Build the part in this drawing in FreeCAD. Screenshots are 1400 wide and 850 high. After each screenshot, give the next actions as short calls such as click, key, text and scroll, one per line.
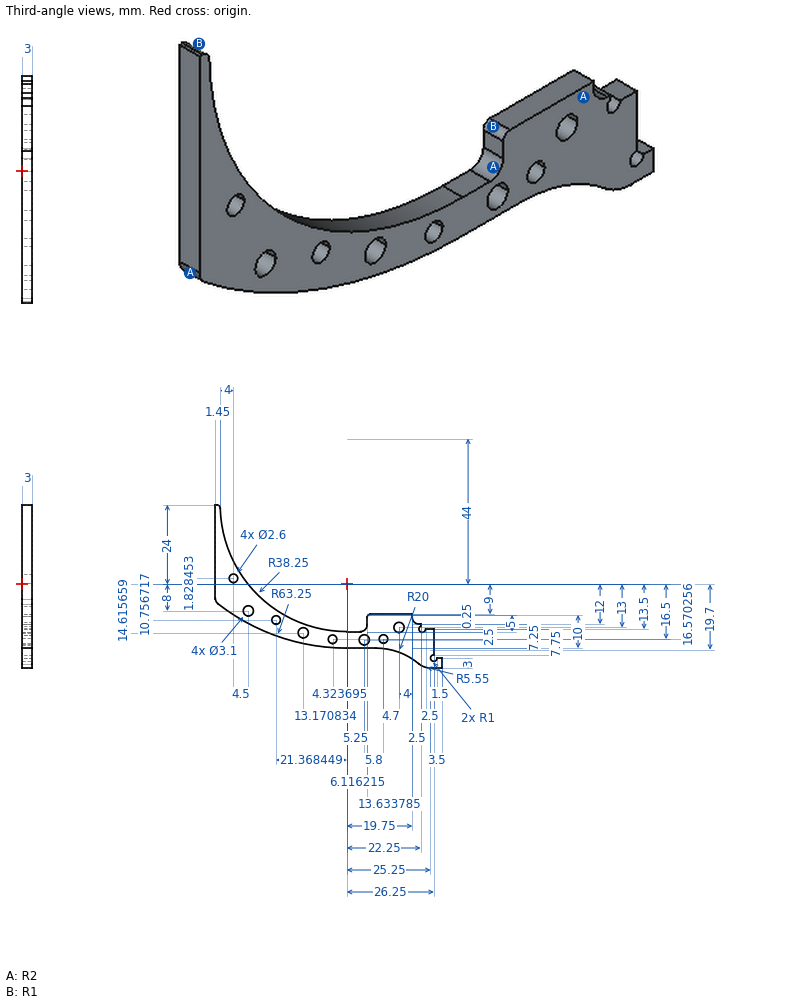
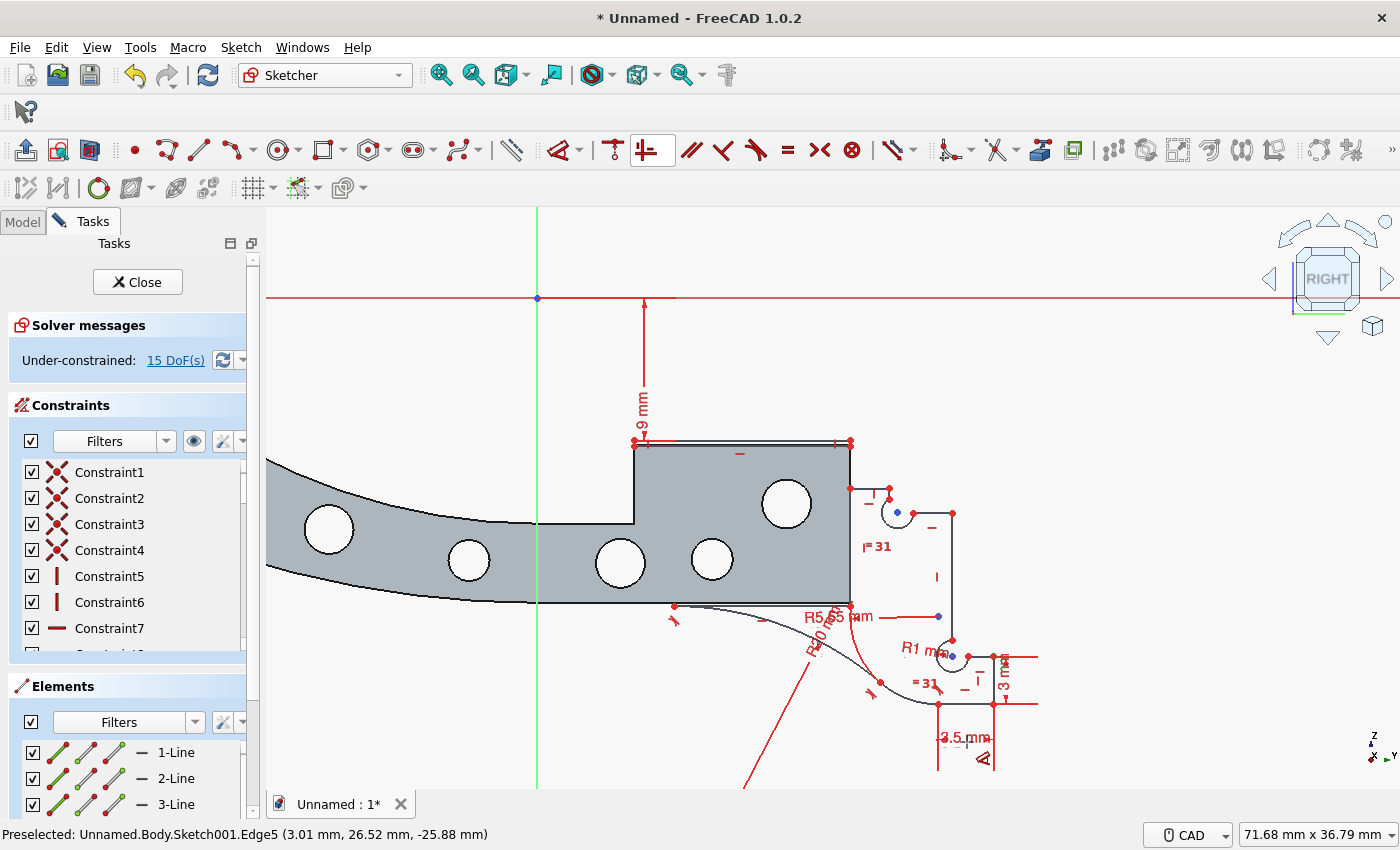
scroll(983, 657, up, 3)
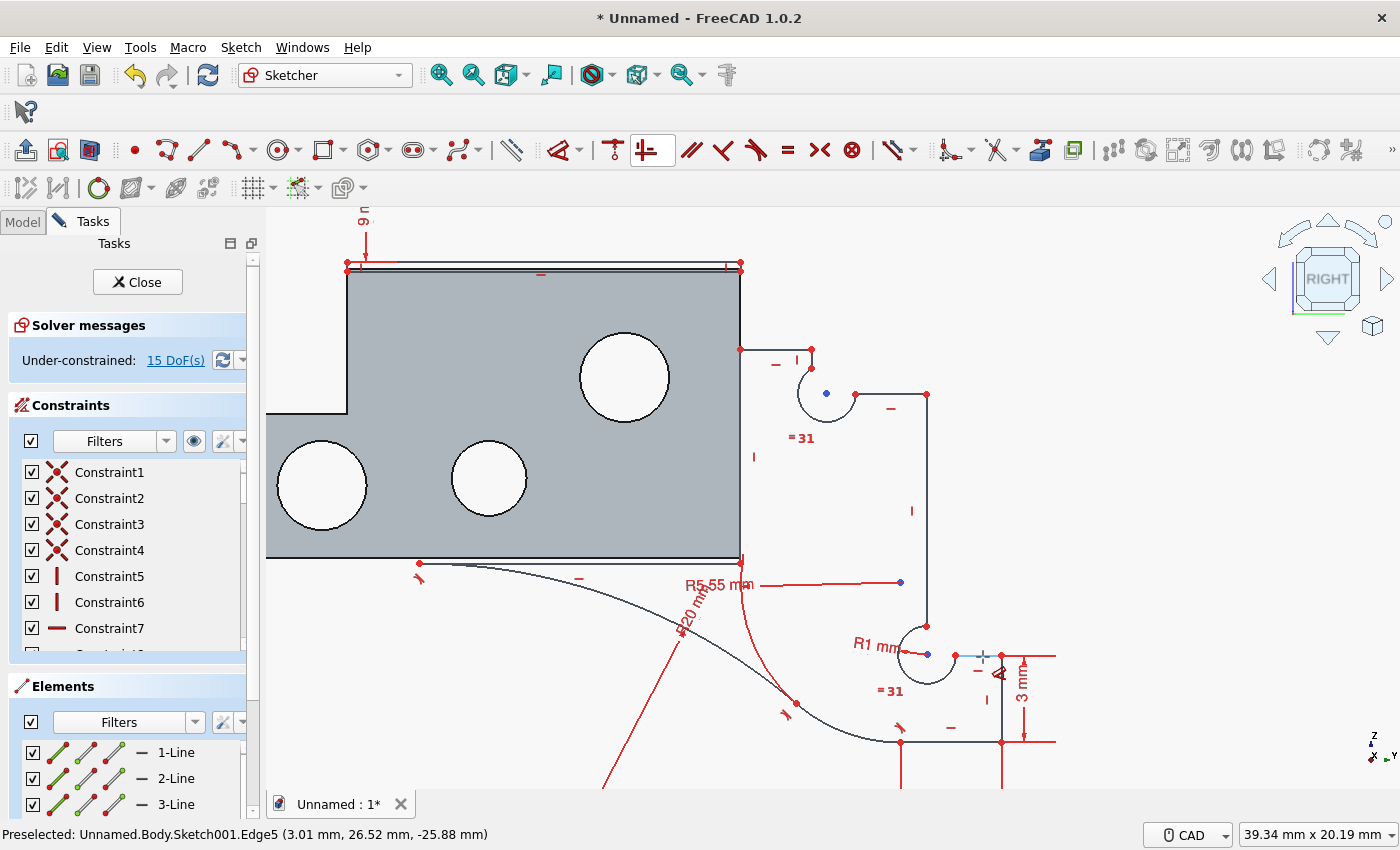
click(983, 656)
click(979, 622)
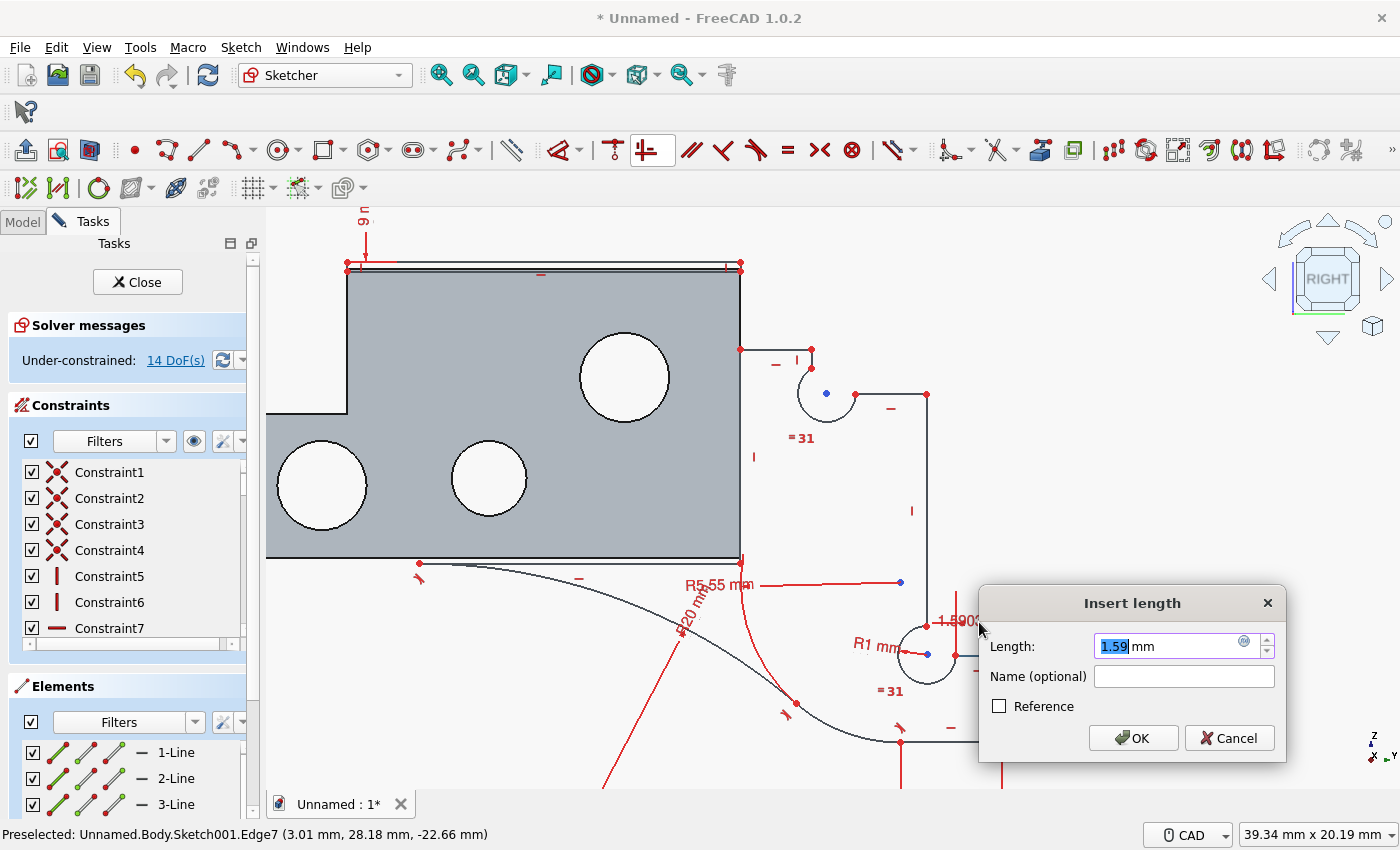
text(1.5)
key(Return)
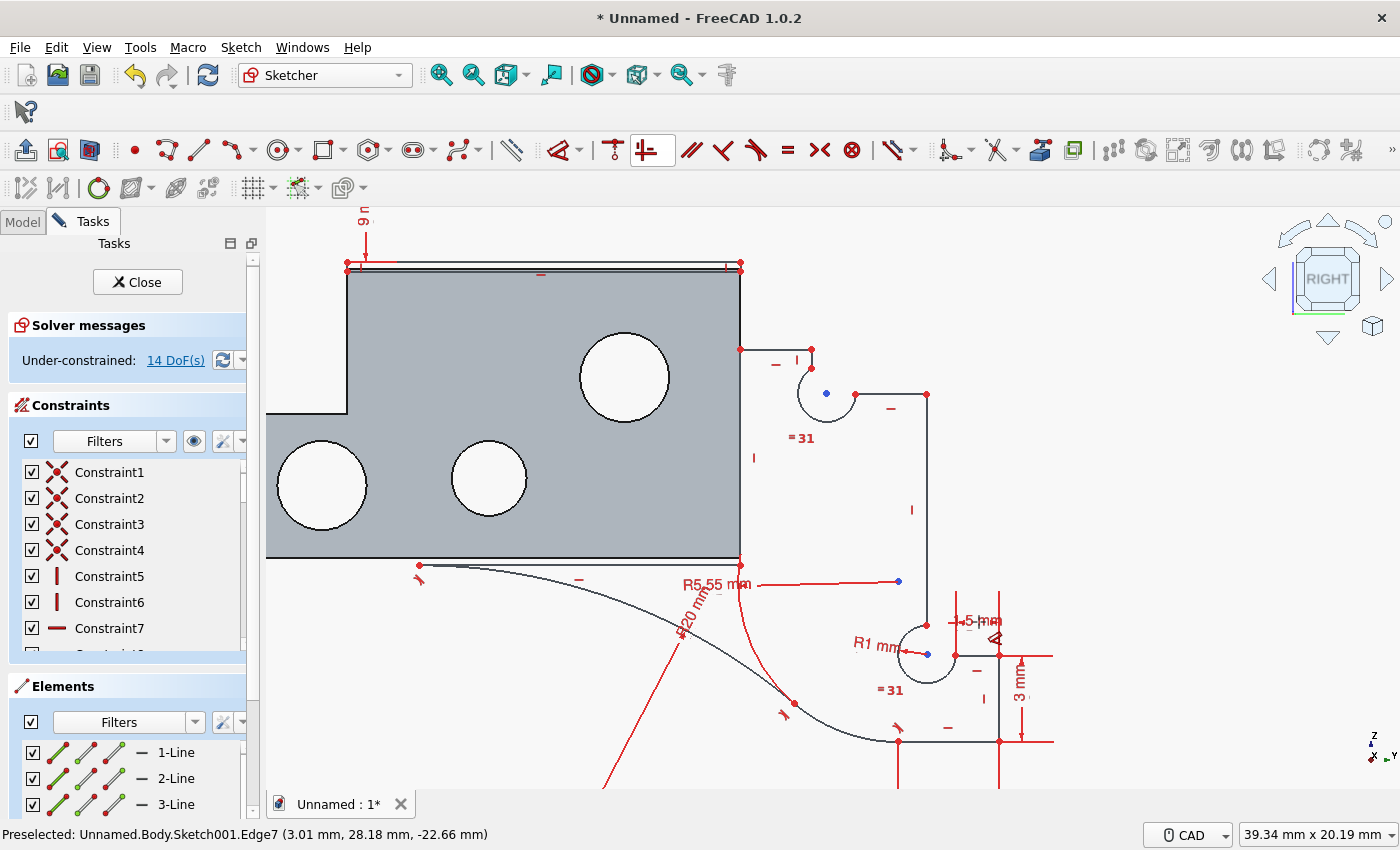
click(905, 394)
click(891, 428)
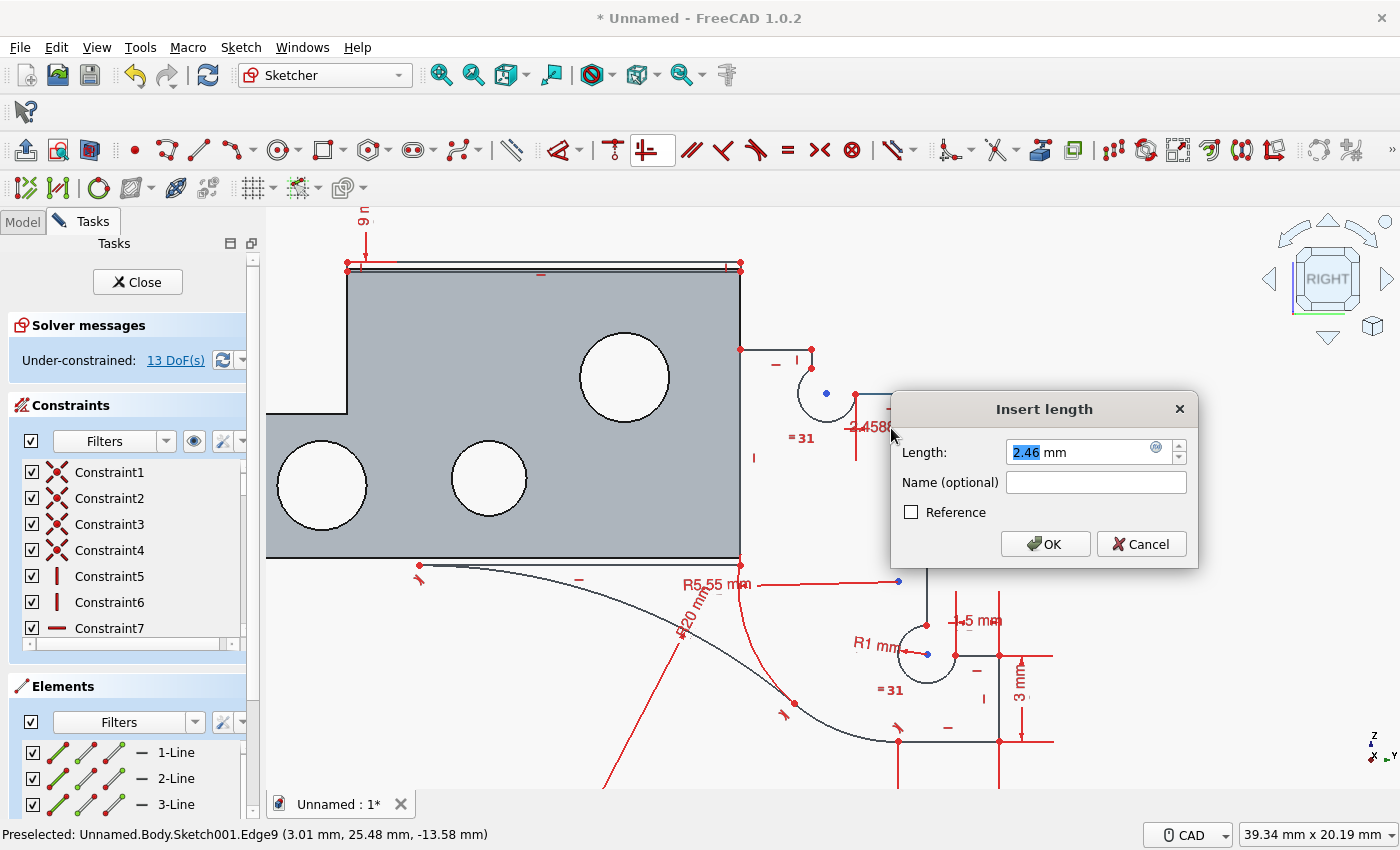
text(2.5)
key(Return)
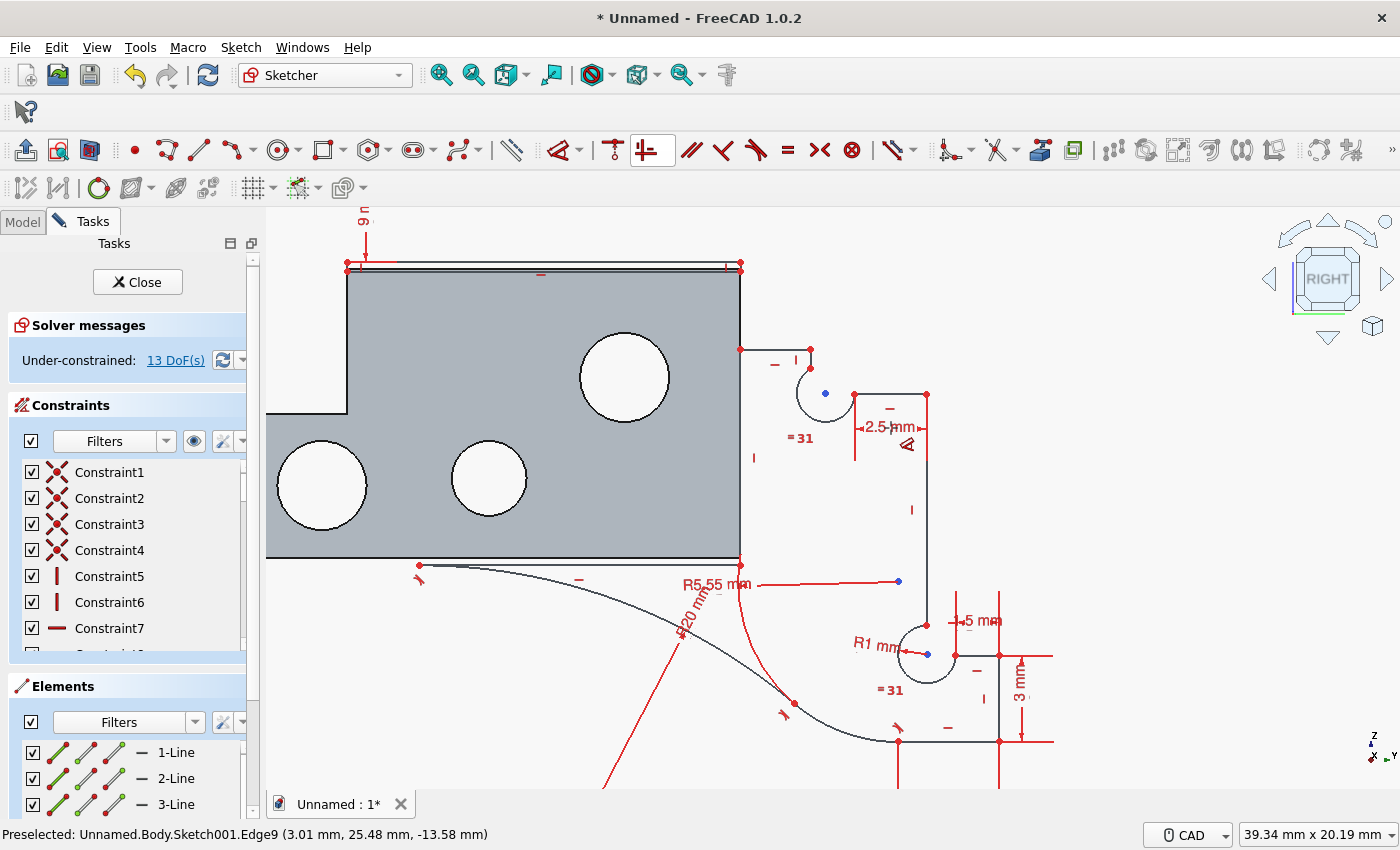
click(789, 350)
click(775, 316)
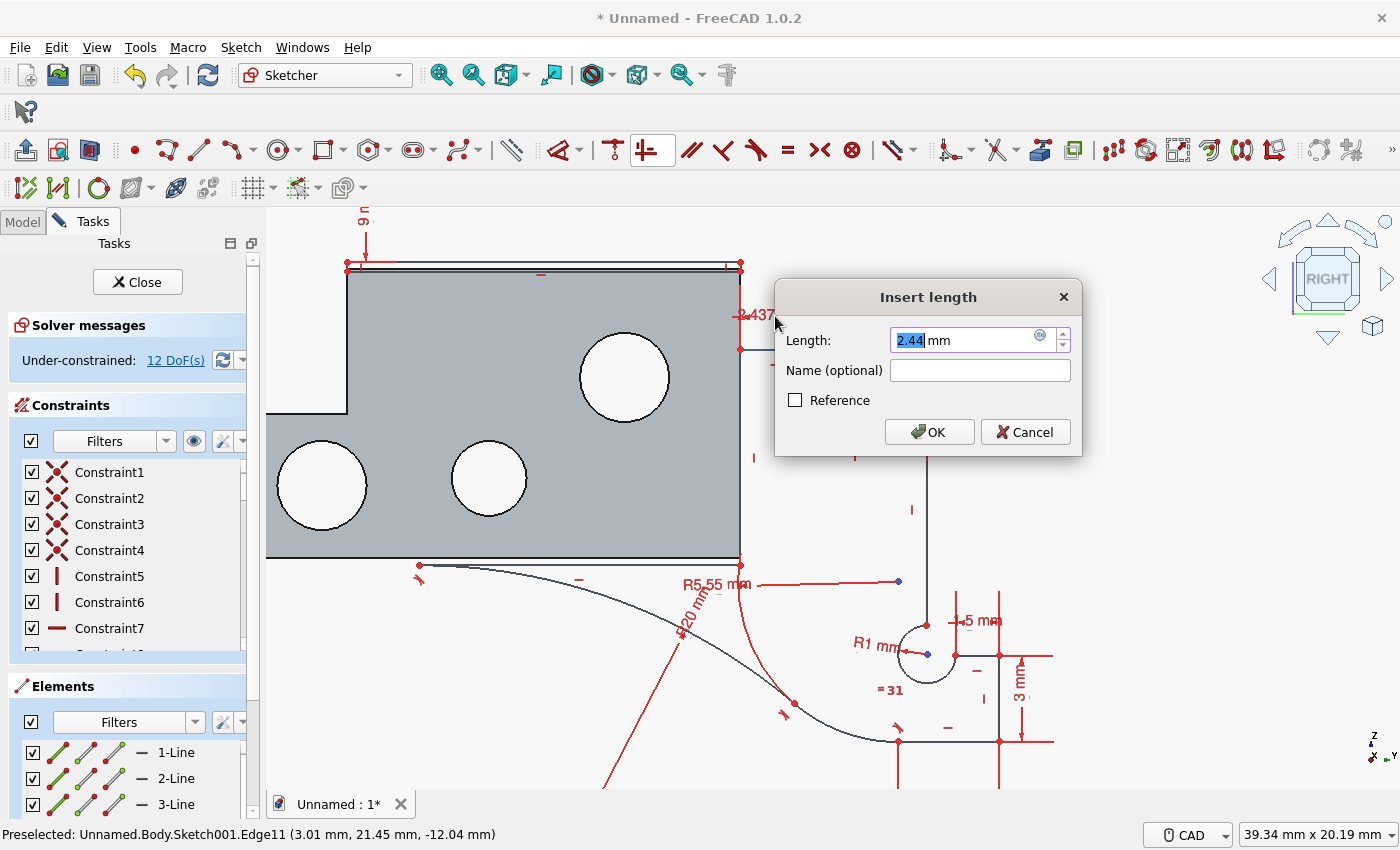
text(2.5)
key(Return)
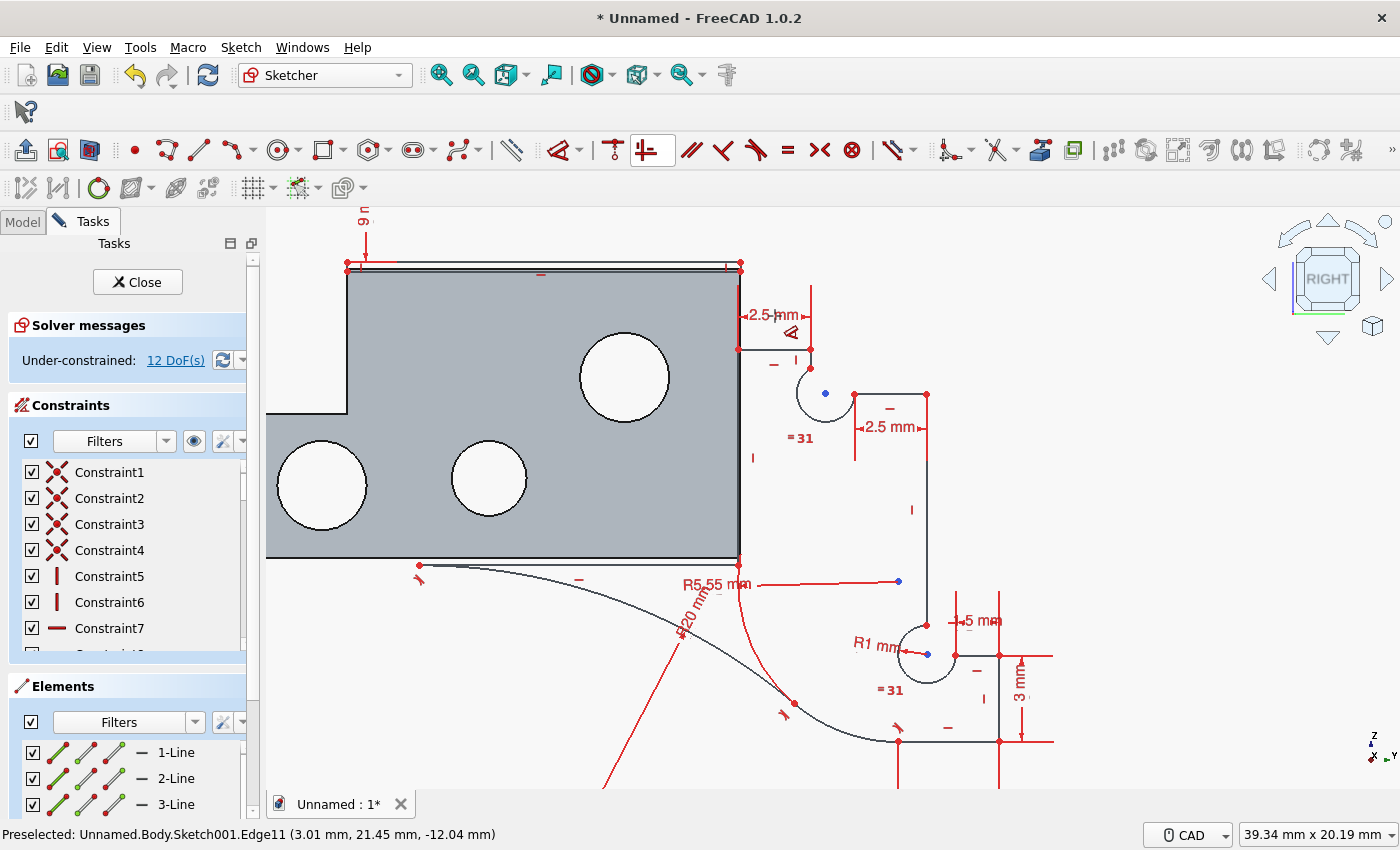
click(811, 350)
click(845, 292)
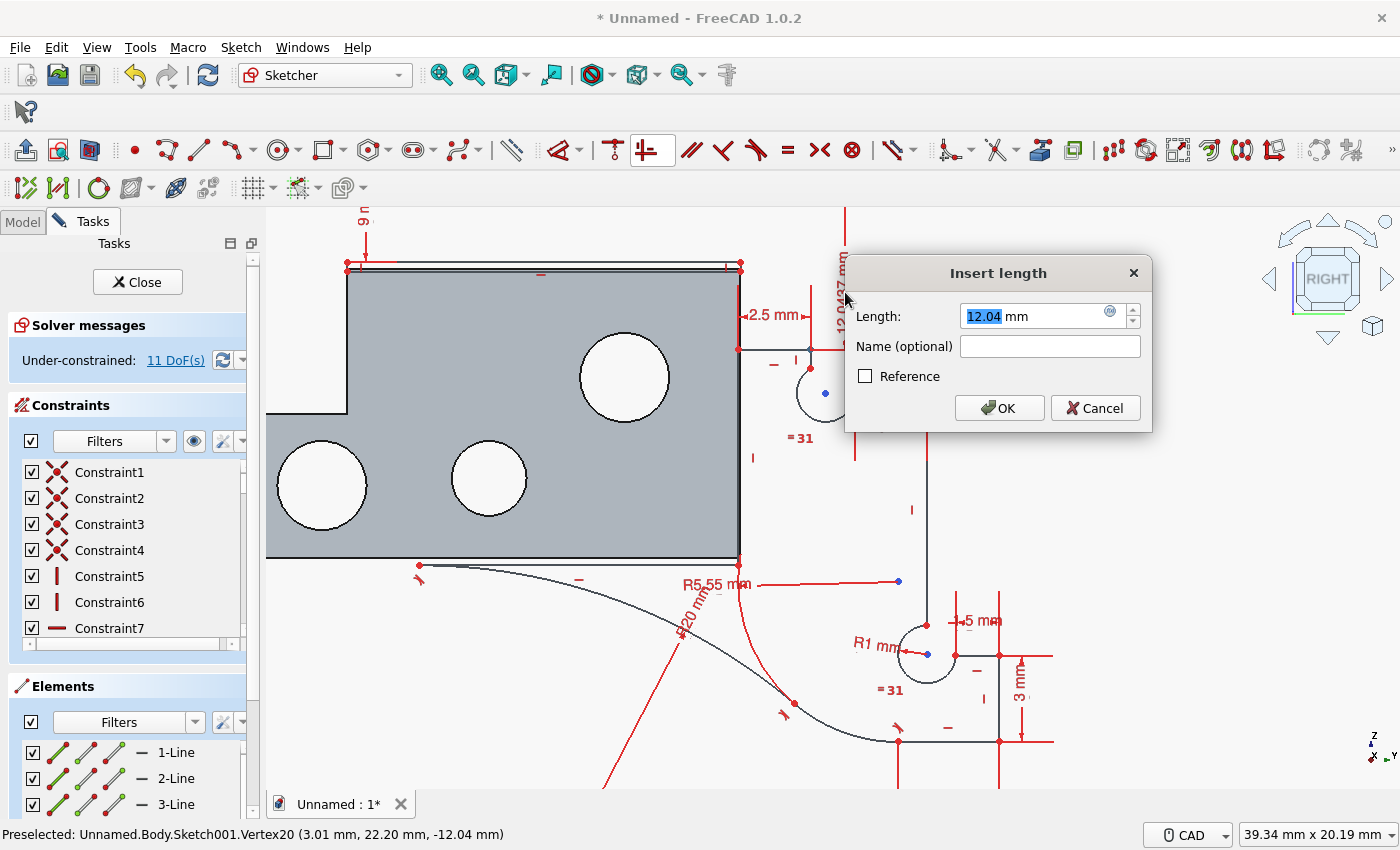
text(12)
key(Return)